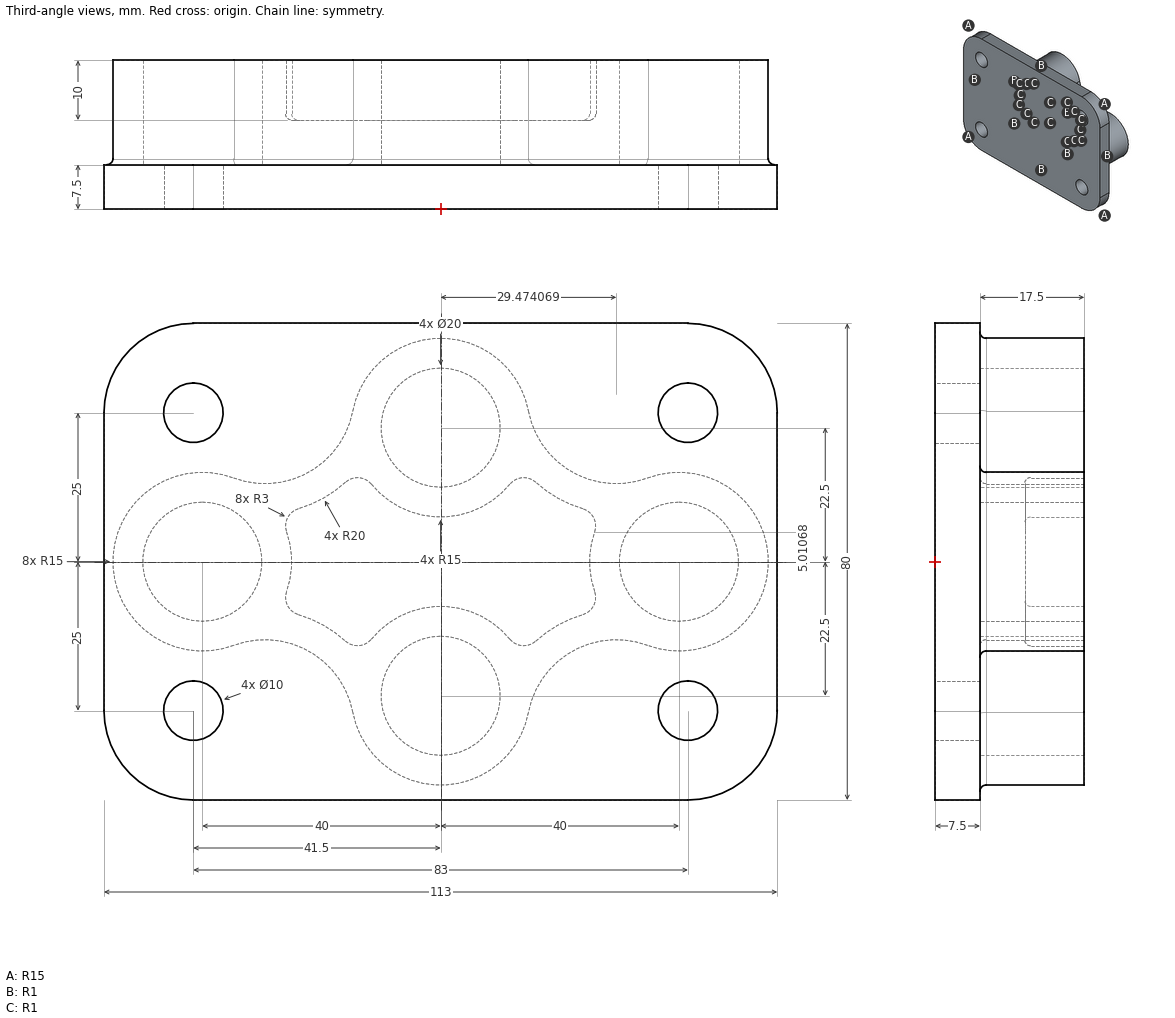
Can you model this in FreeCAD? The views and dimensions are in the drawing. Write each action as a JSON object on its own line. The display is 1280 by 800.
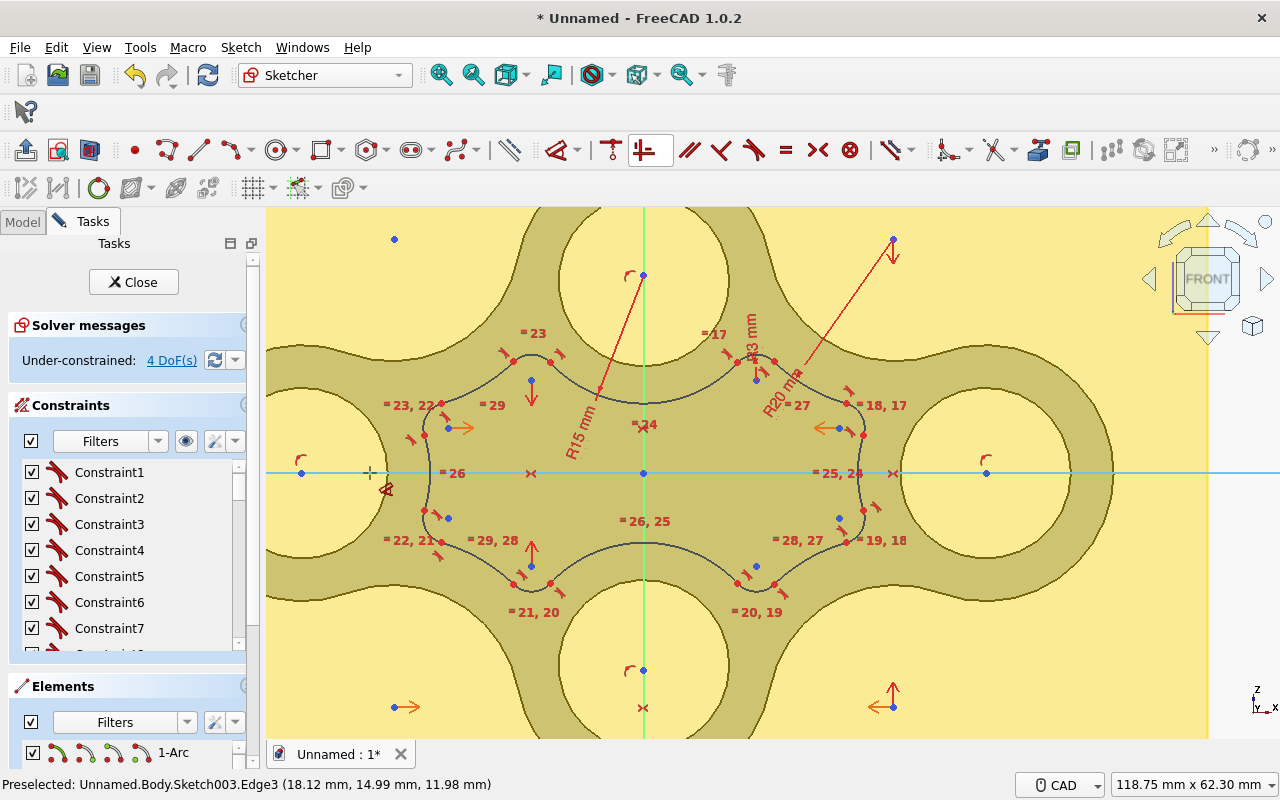
{"action": "left_click", "coordinate": [986, 473]}
{"action": "left_click", "coordinate": [815, 507]}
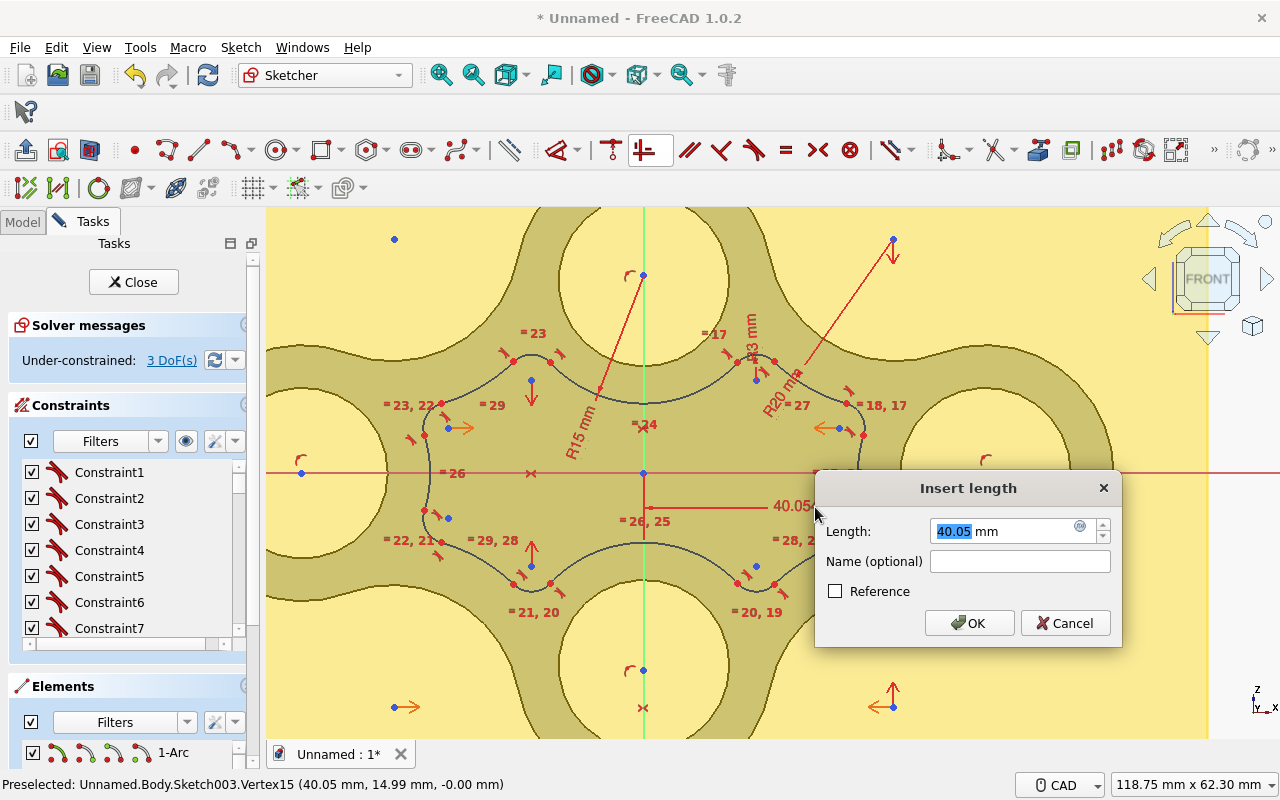
{"action": "type", "text": "40"}
{"action": "key", "text": "Return"}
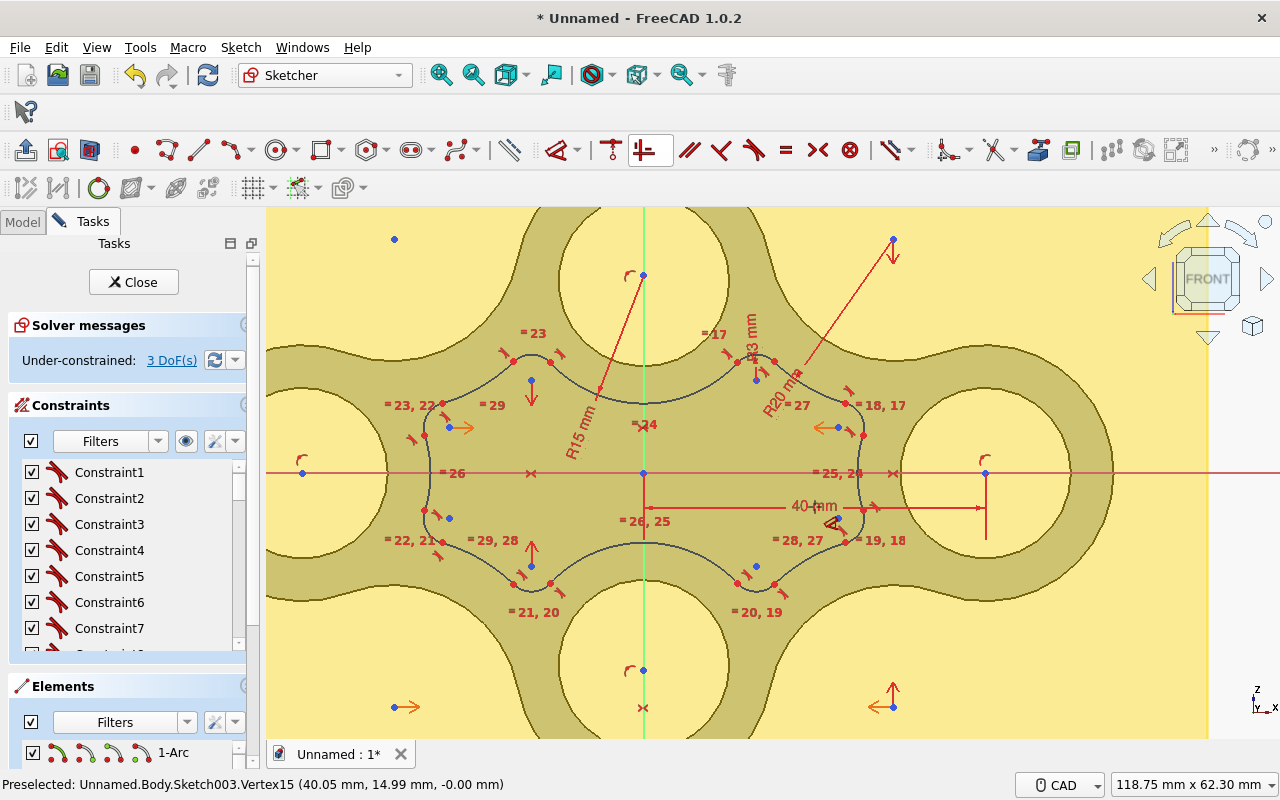
{"action": "left_click", "coordinate": [644, 275]}
{"action": "left_click", "coordinate": [678, 374]}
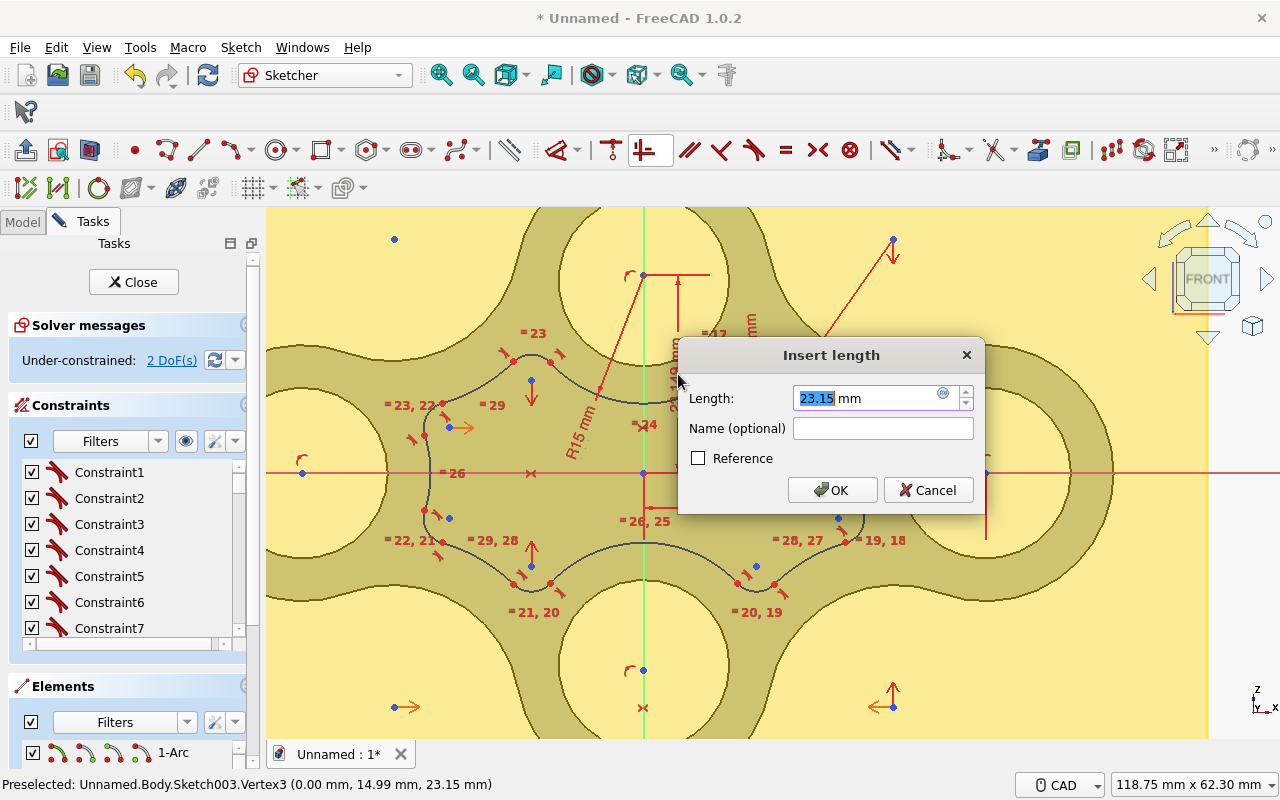
{"action": "type", "text": "22.5"}
{"action": "key", "text": "Return"}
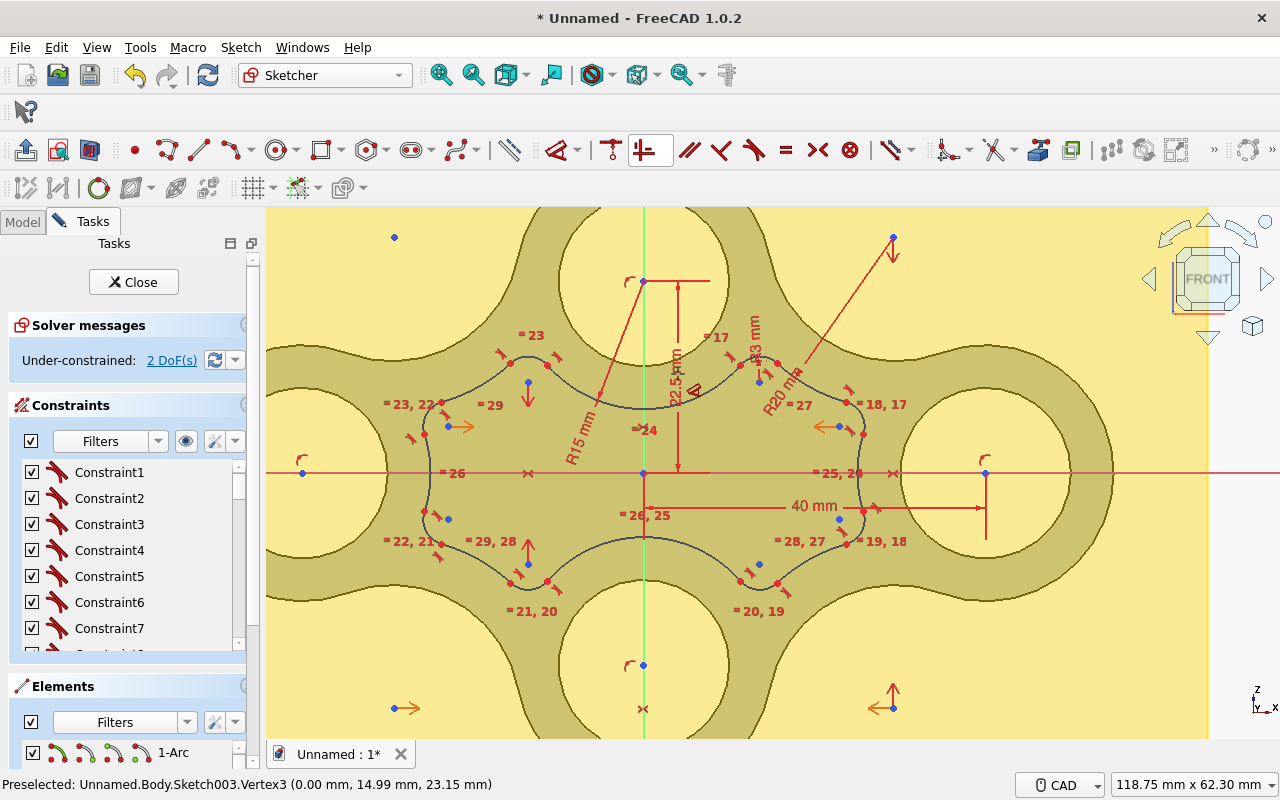
{"action": "left_click", "coordinate": [863, 434]}
{"action": "left_click", "coordinate": [897, 454]}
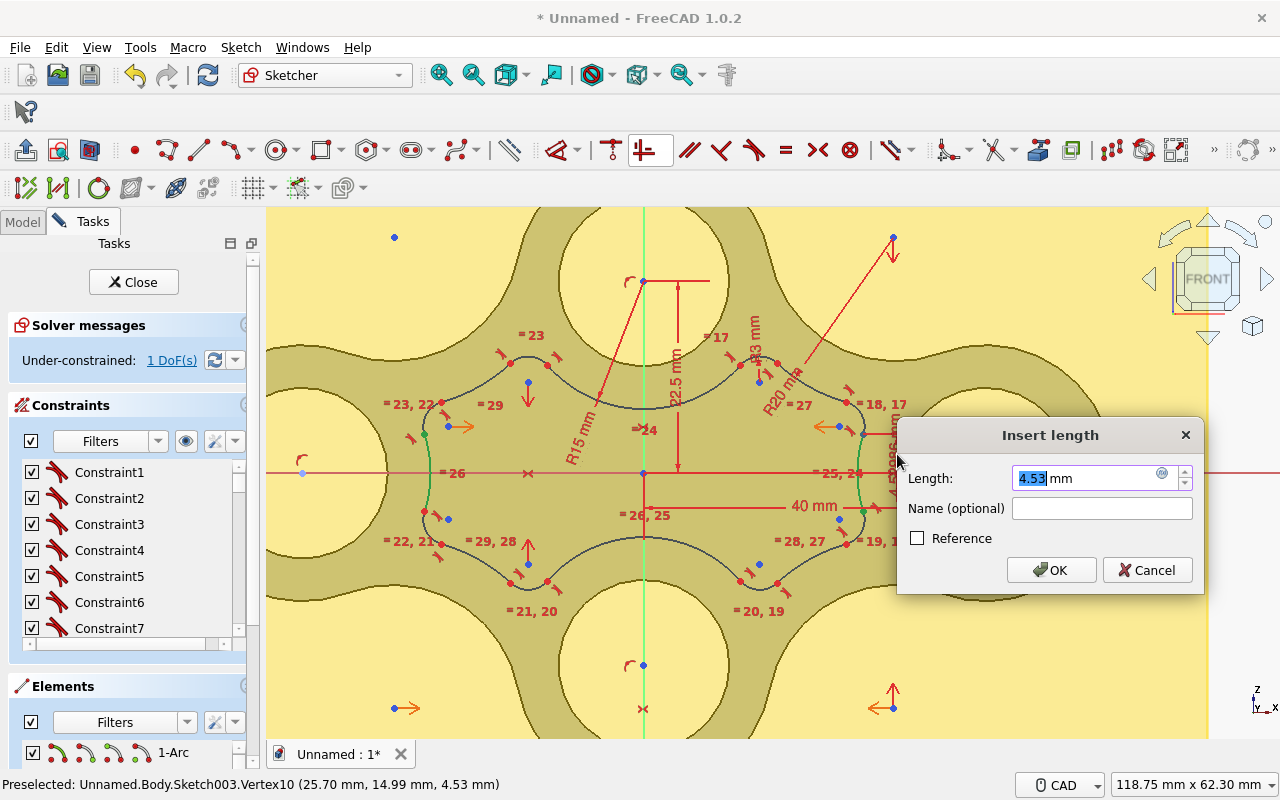
{"action": "type", "text": "5.01068"}
{"action": "key", "text": "Return"}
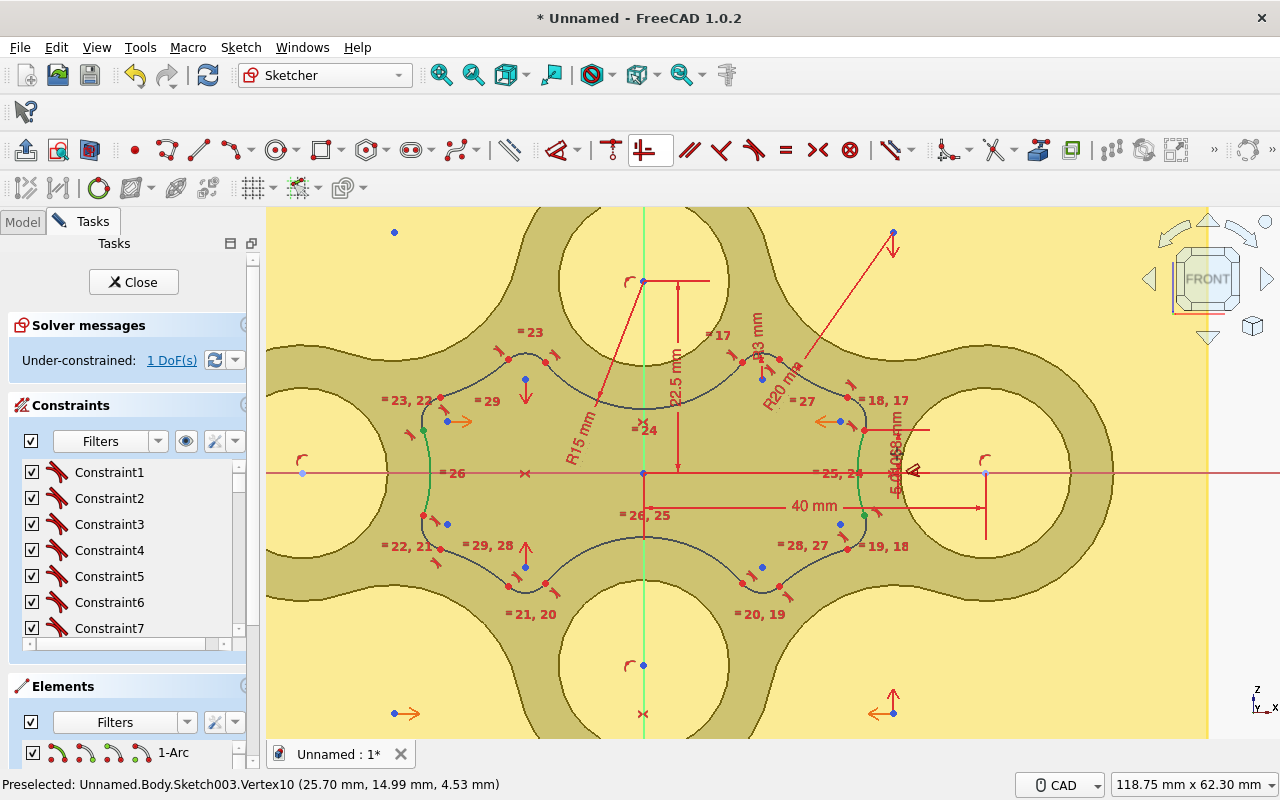
{"action": "scroll", "coordinate": [914, 711], "scroll_direction": "down", "scroll_amount": 1}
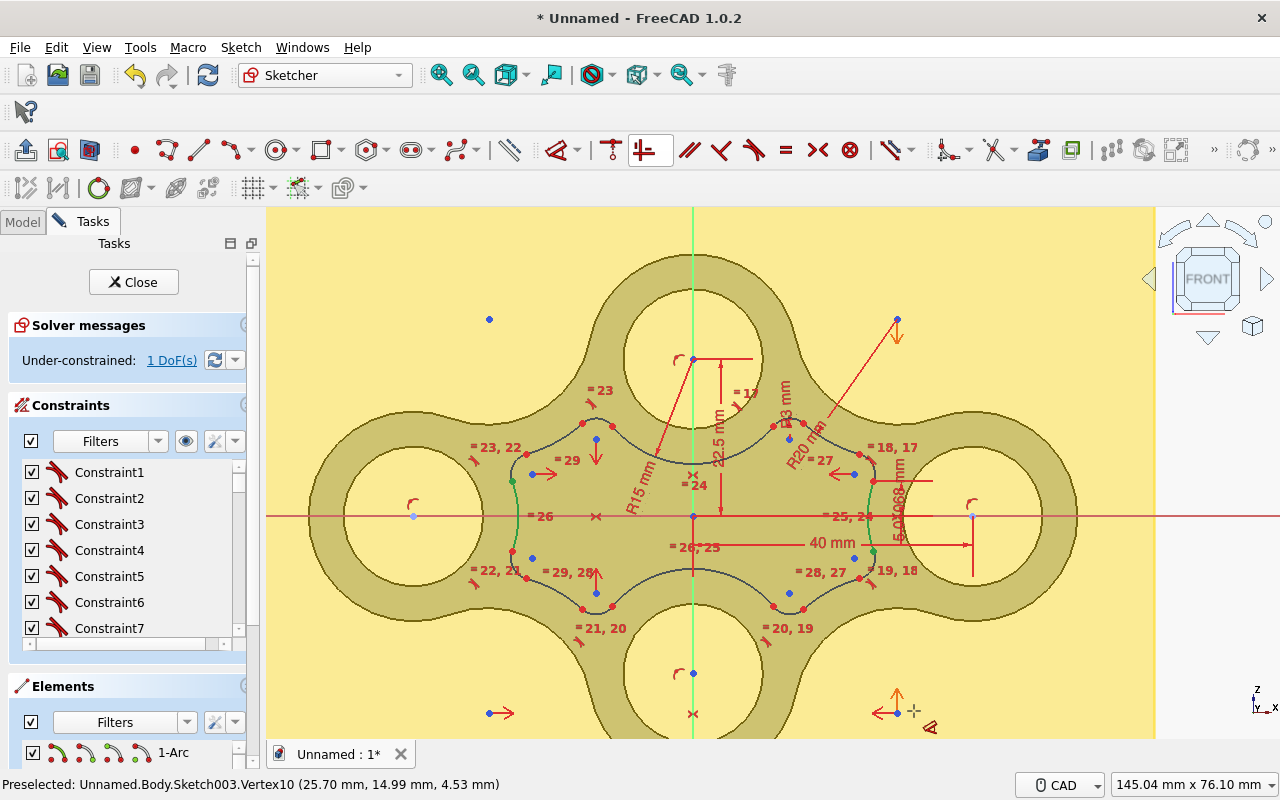
{"action": "left_click", "coordinate": [897, 319]}
{"action": "left_click", "coordinate": [795, 285]}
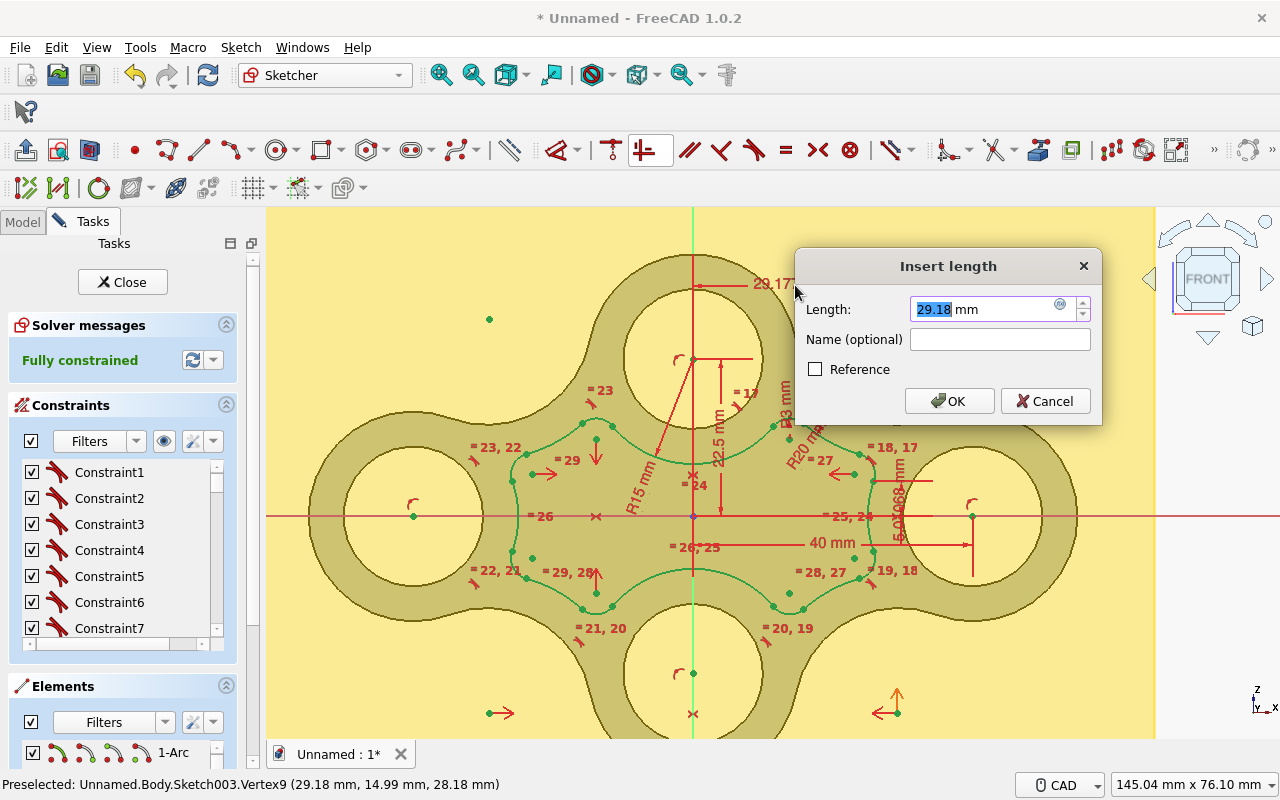
{"action": "type", "text": "29.474069"}
{"action": "key", "text": "Return"}
{"action": "key", "text": "Escape"}